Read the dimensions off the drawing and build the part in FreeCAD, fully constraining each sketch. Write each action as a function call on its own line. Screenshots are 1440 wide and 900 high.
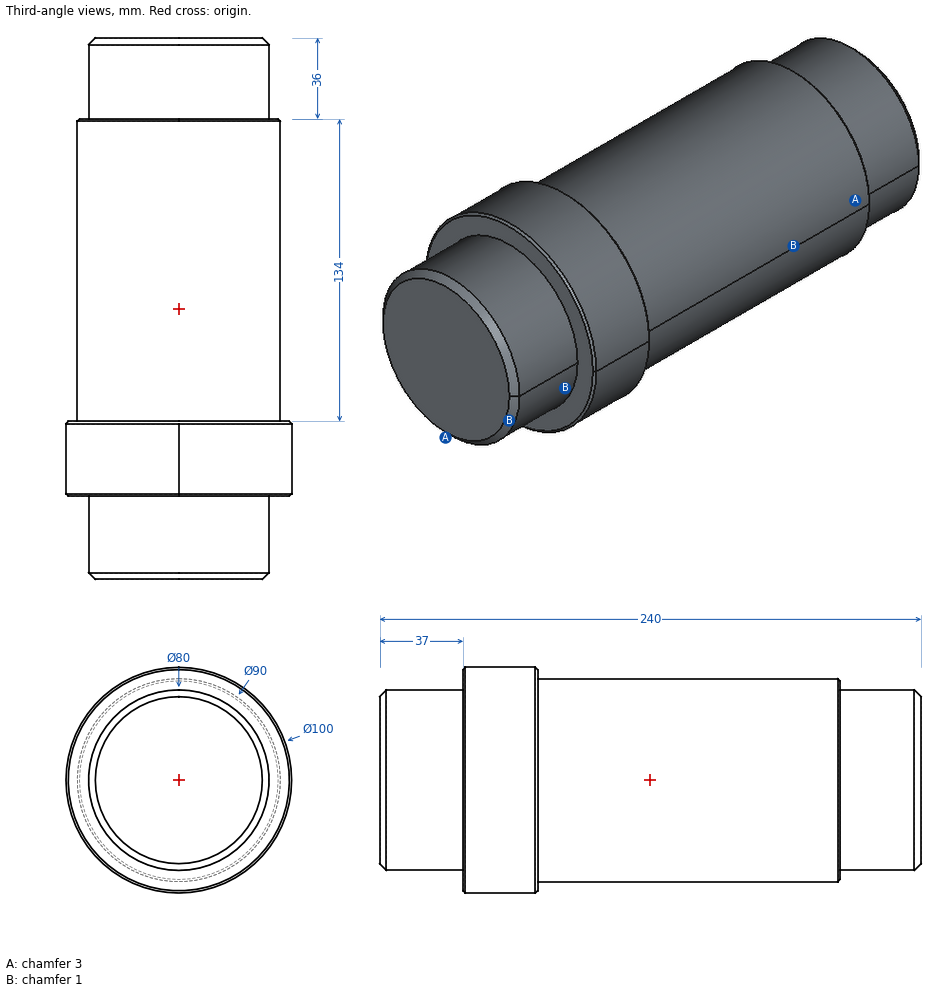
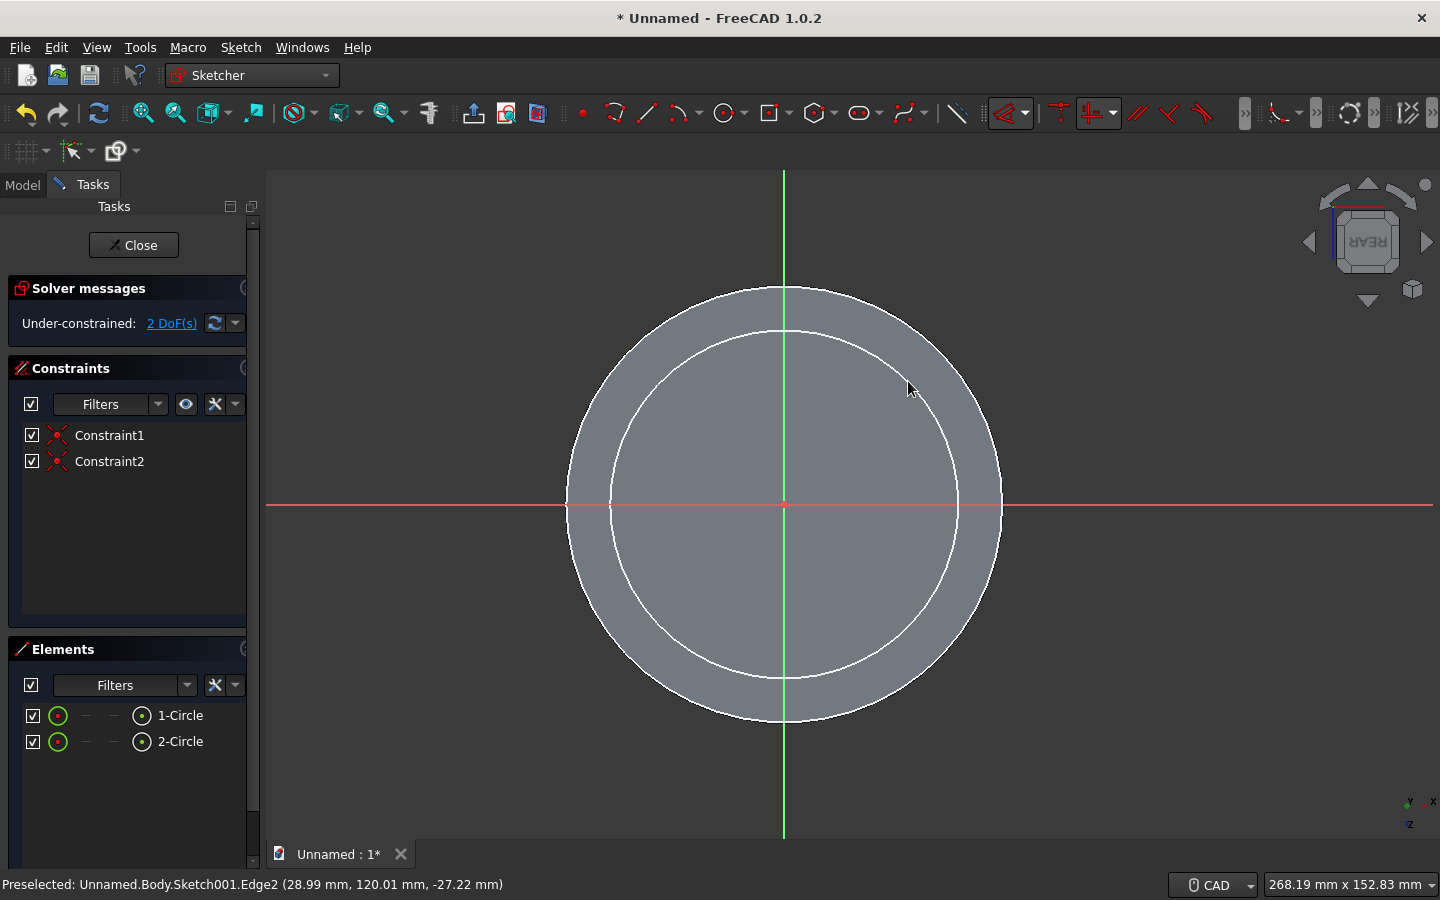
click(1004, 114)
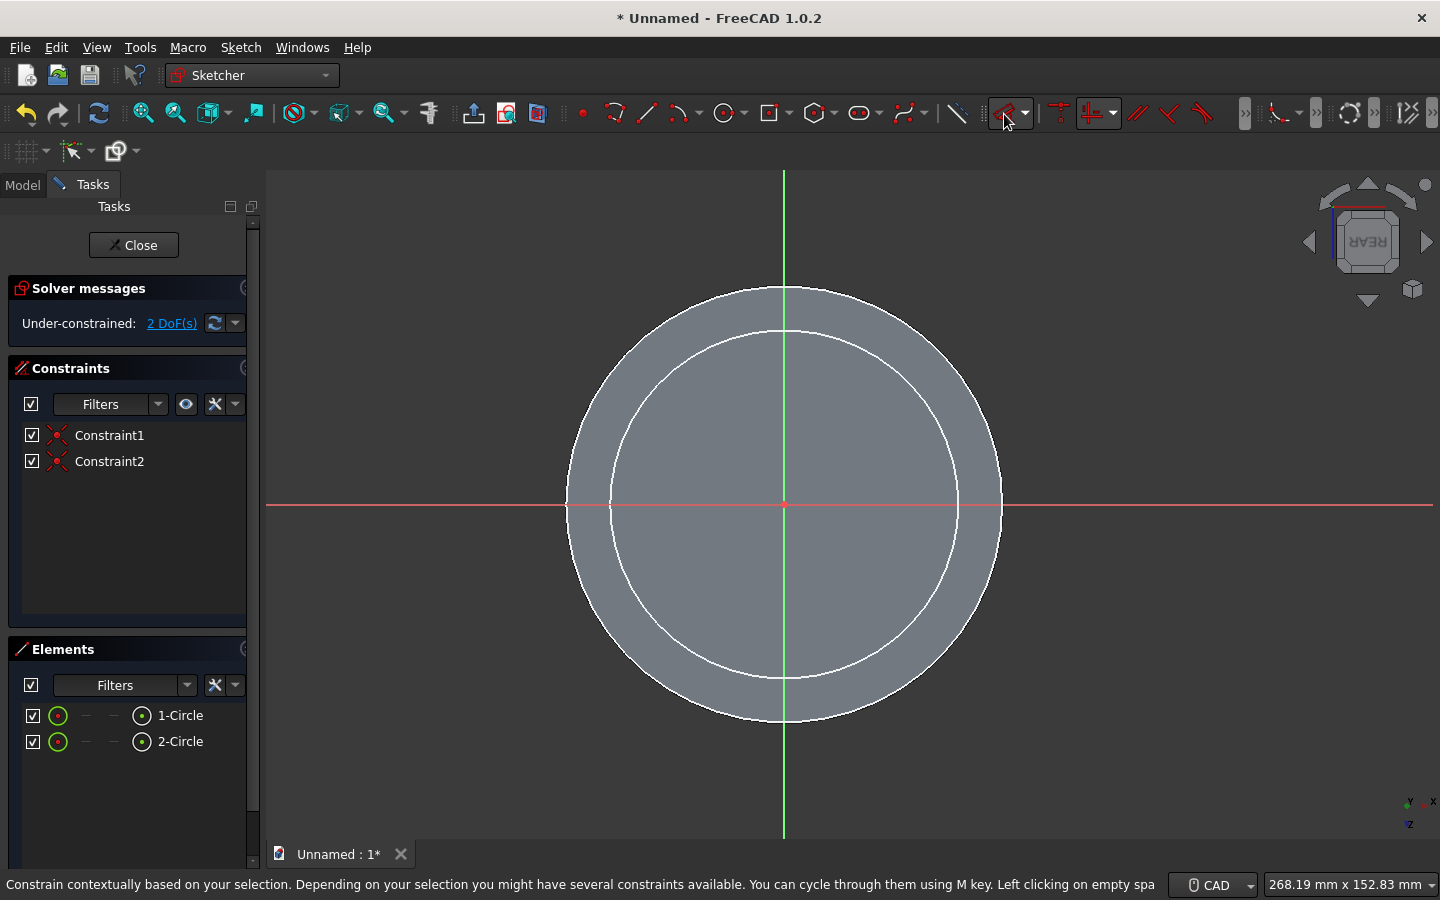
click(938, 350)
click(961, 327)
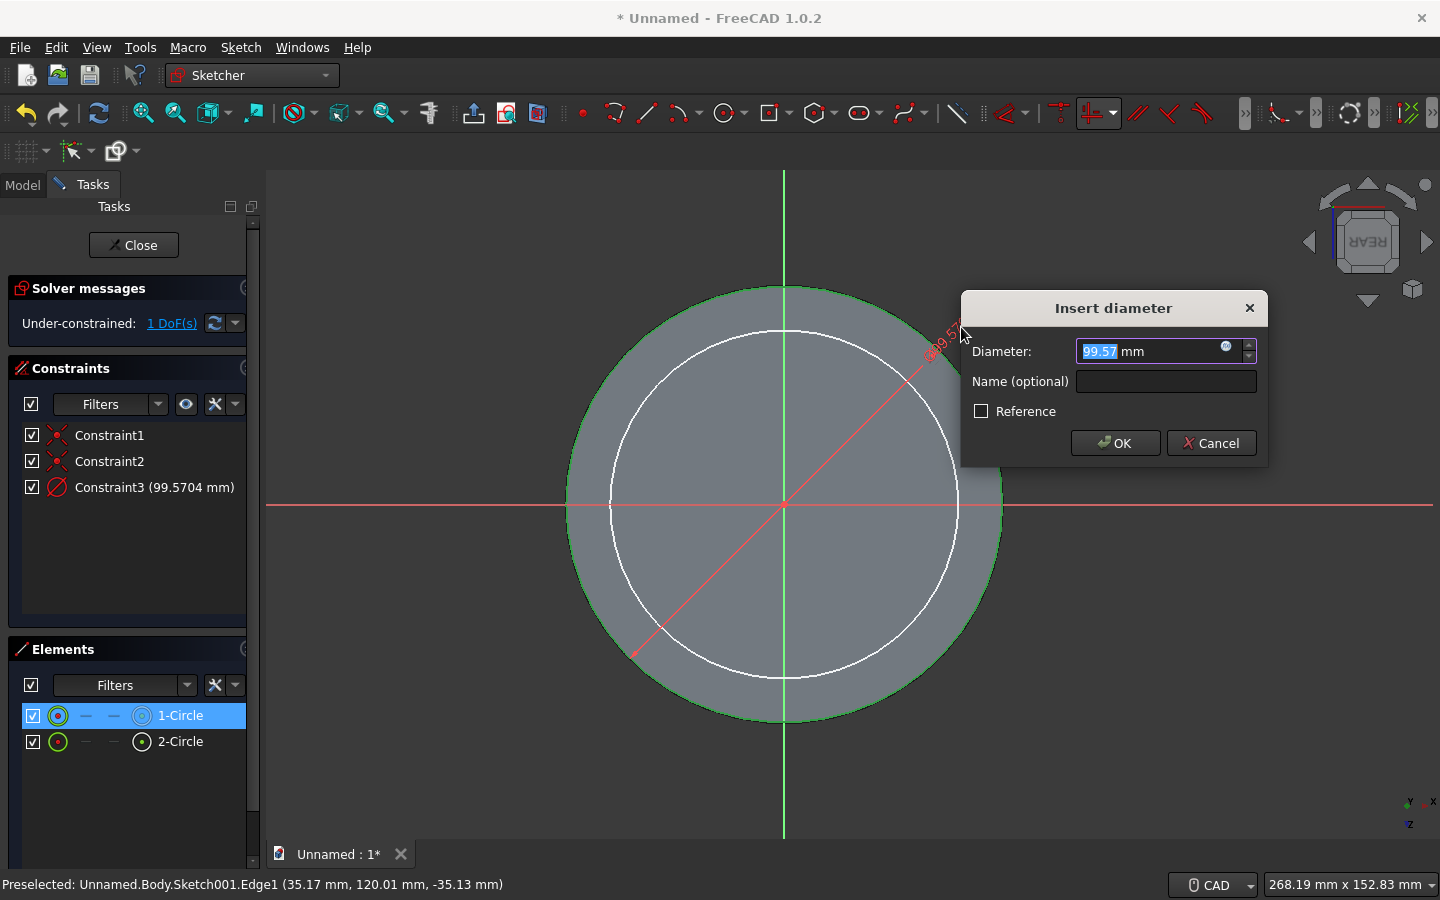
text(100)
key(Return)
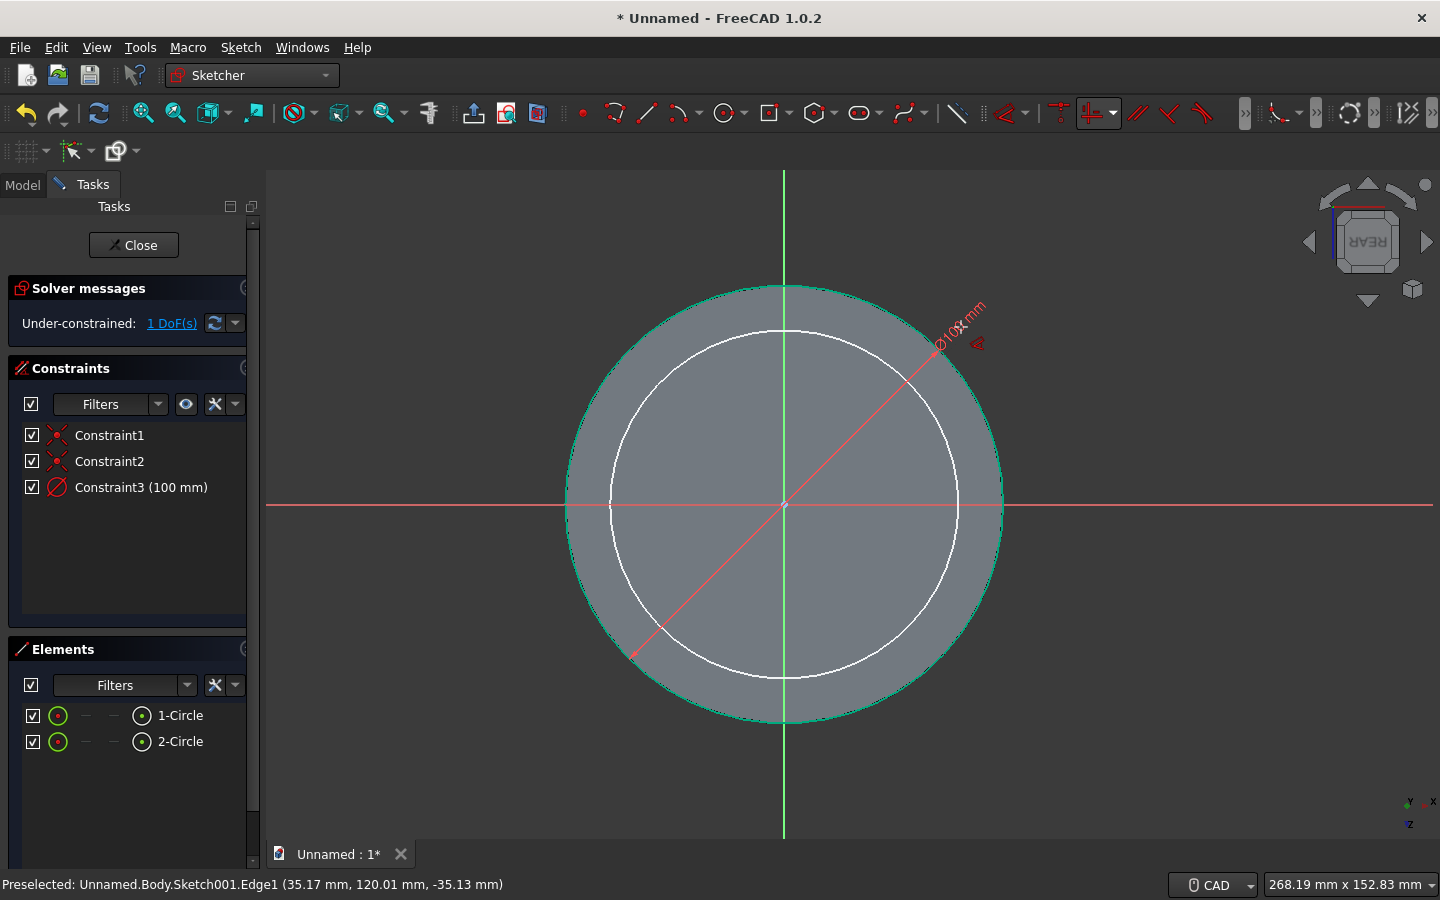
click(907, 381)
click(1028, 432)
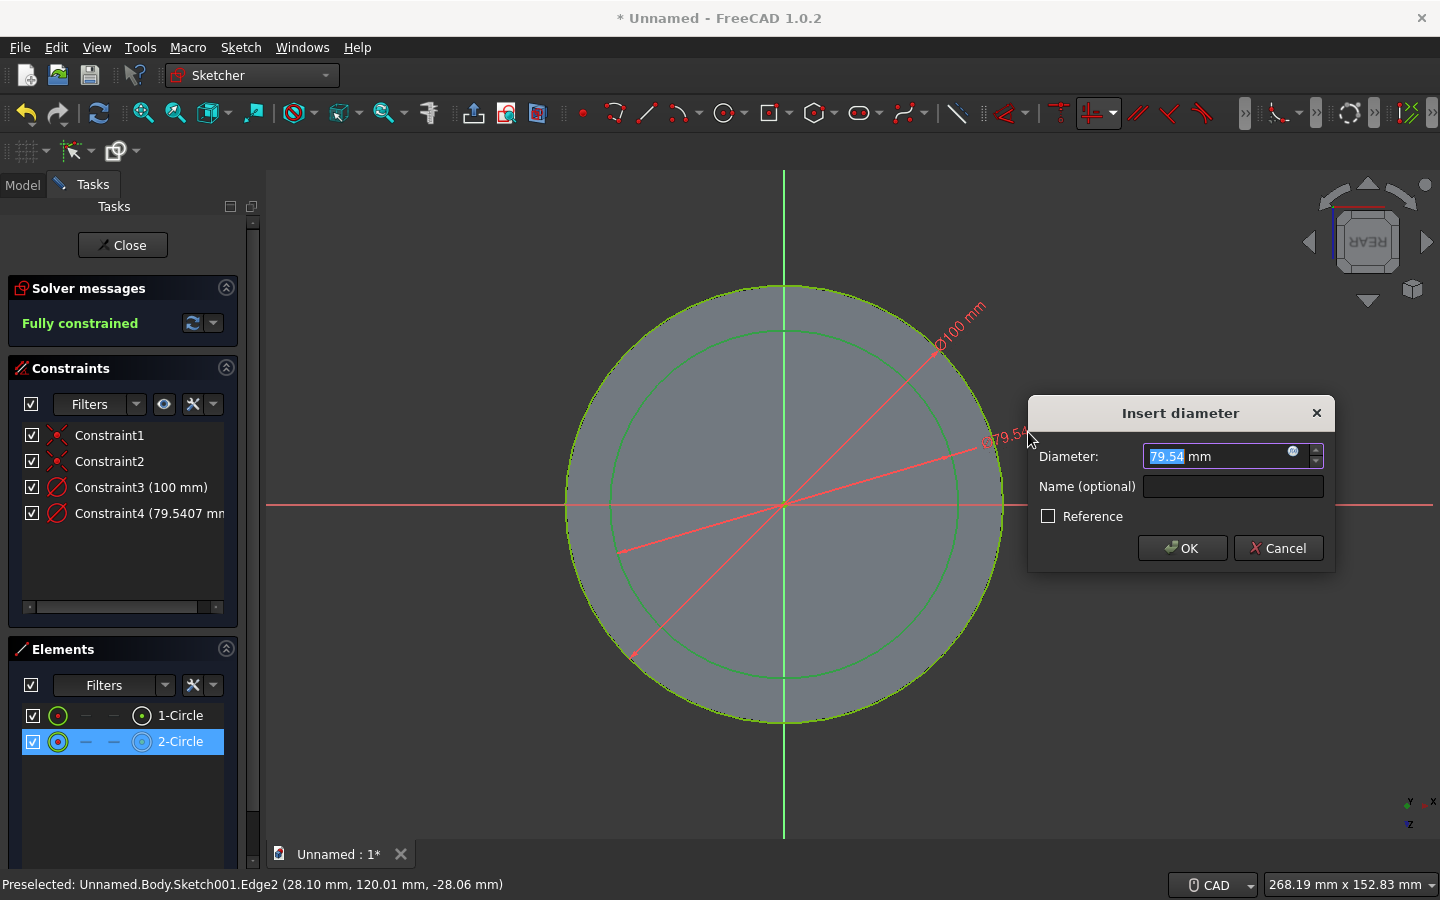
text(80)
key(Return)
key(Escape)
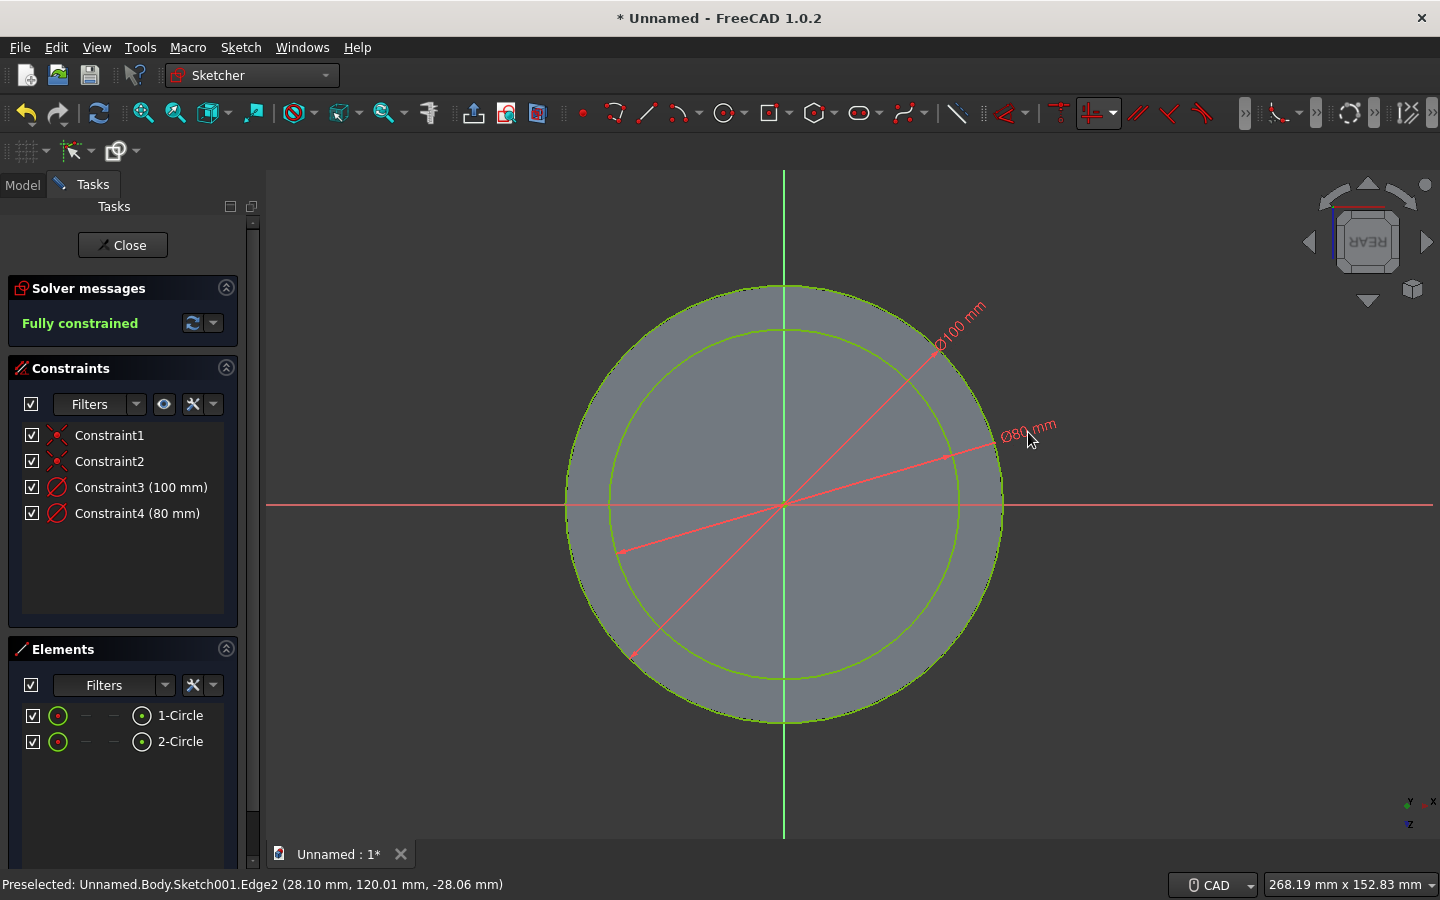
click(123, 245)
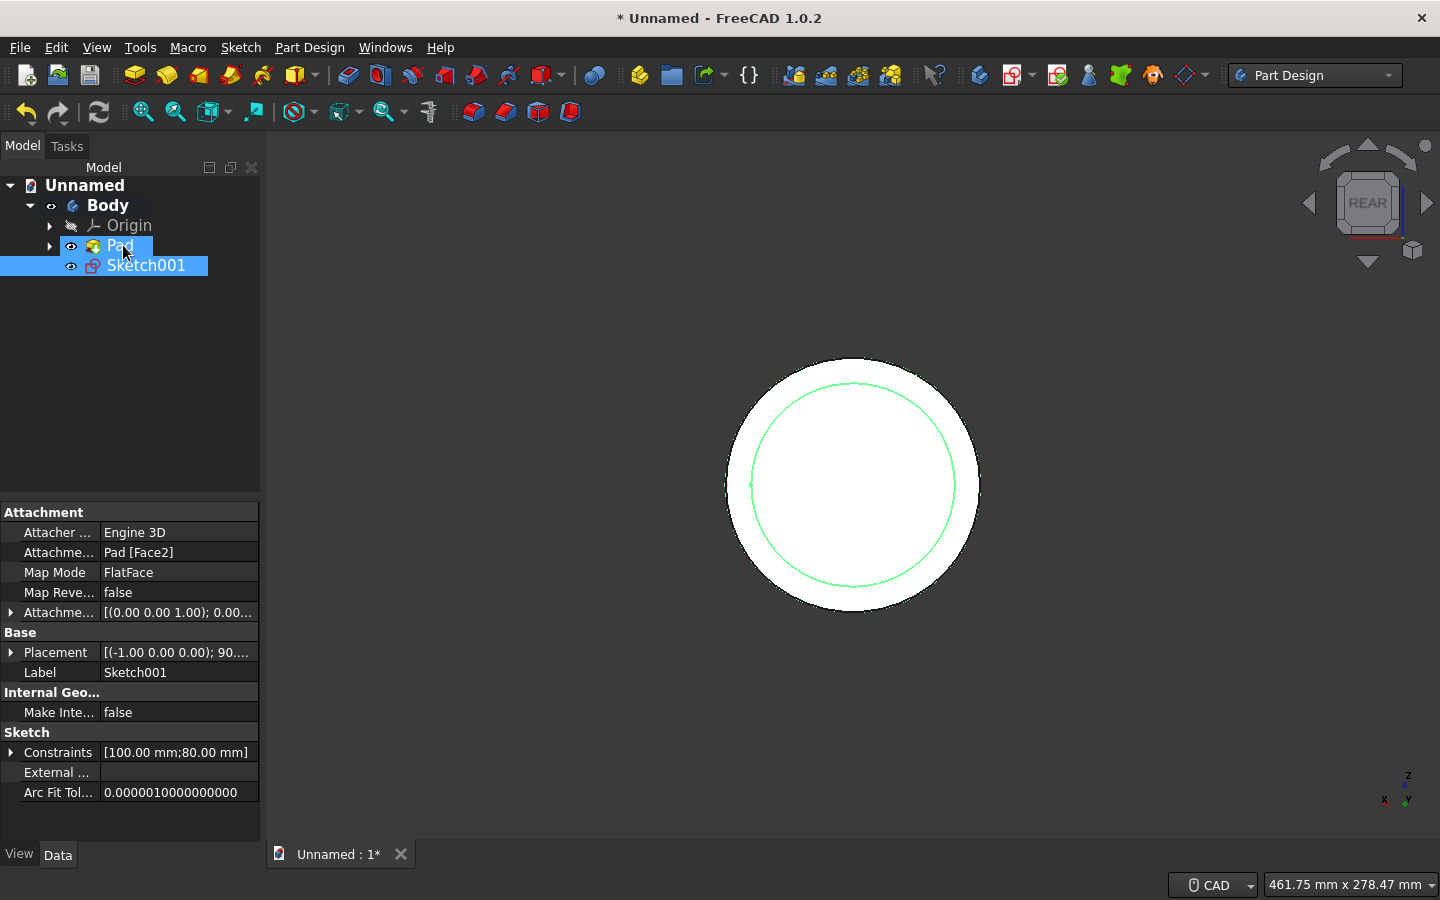
click(350, 76)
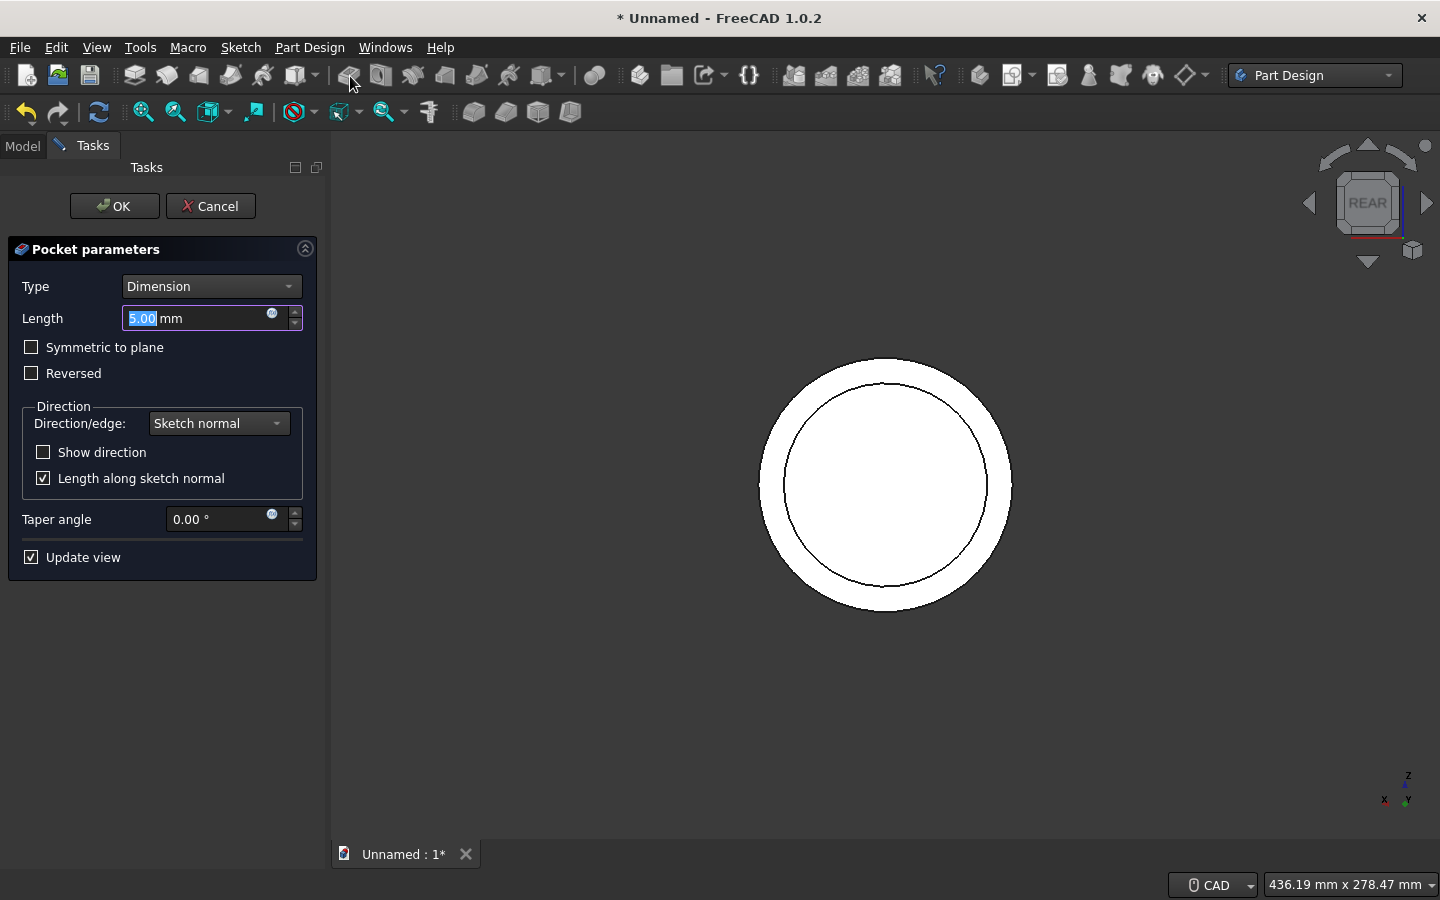
text(36)
key(Tab)